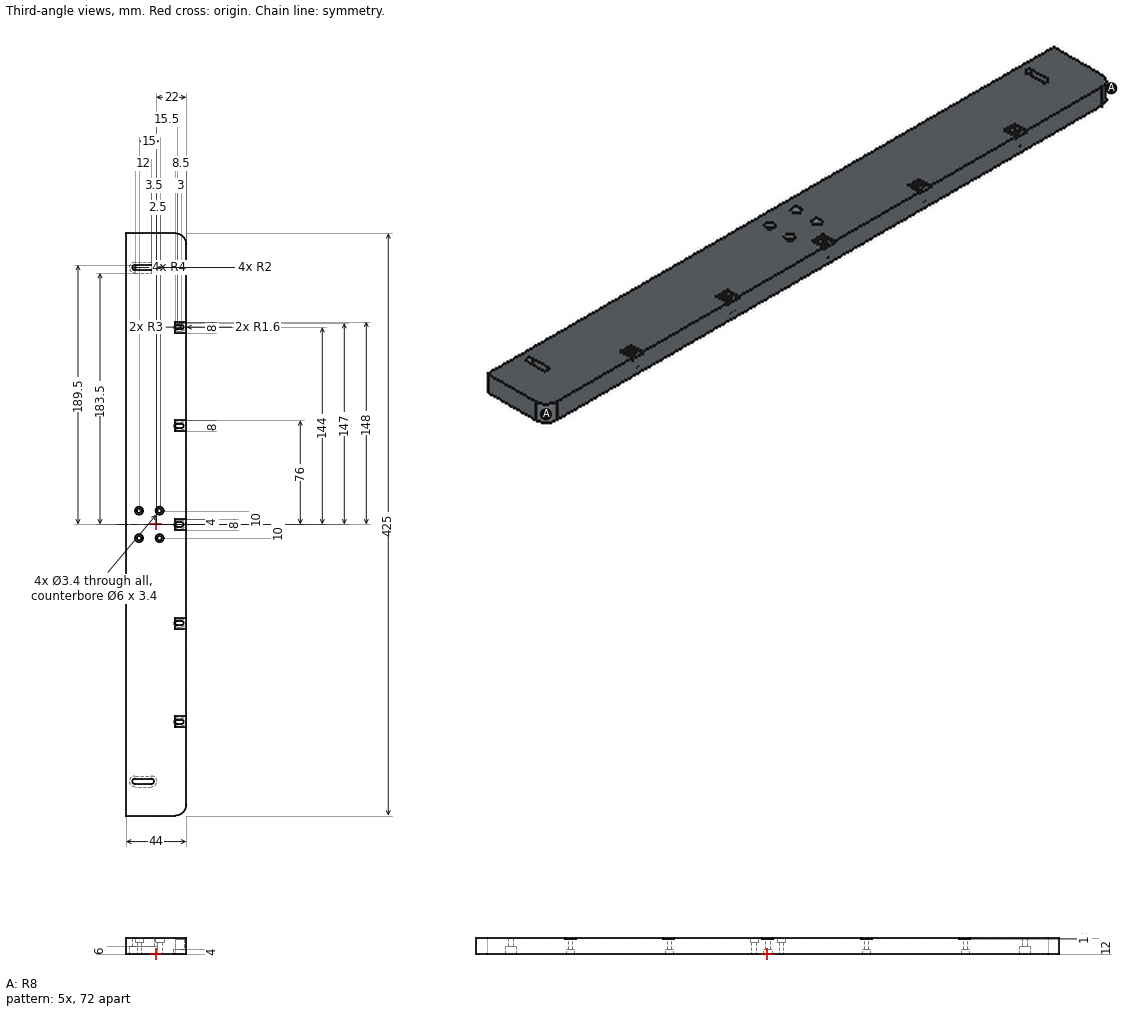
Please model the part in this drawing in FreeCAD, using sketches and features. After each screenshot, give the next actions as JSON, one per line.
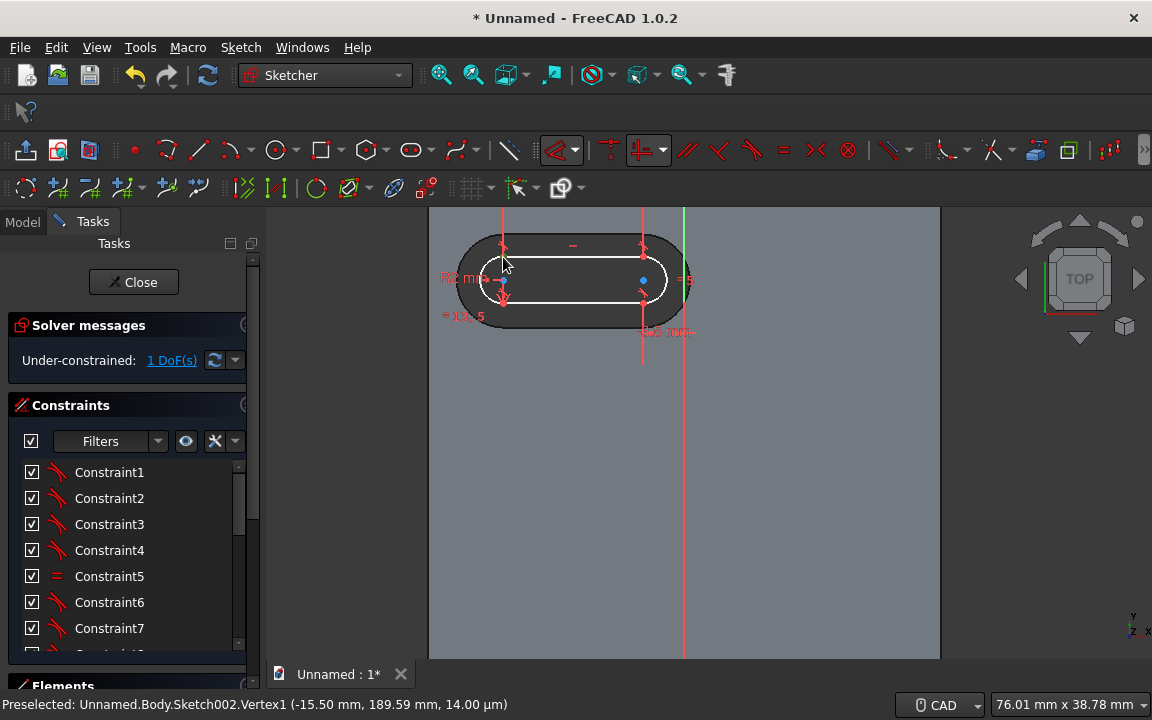
{"action": "key", "text": "i"}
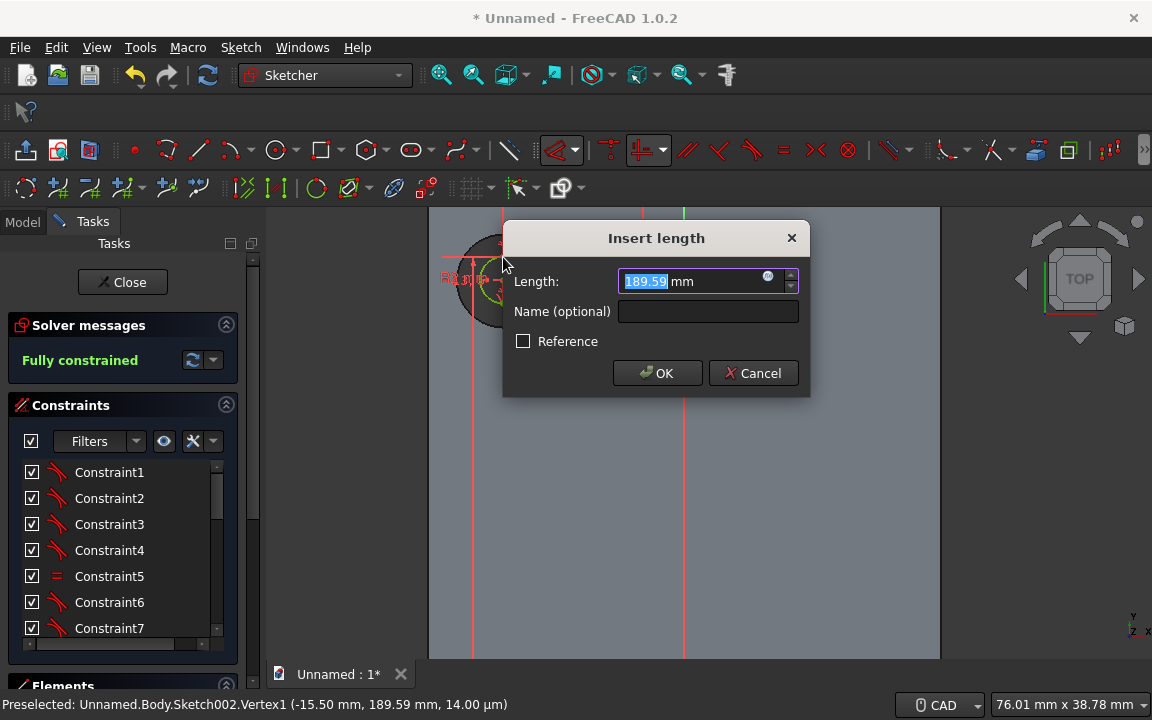
{"action": "type", "text": "189.5"}
{"action": "key", "text": "Return"}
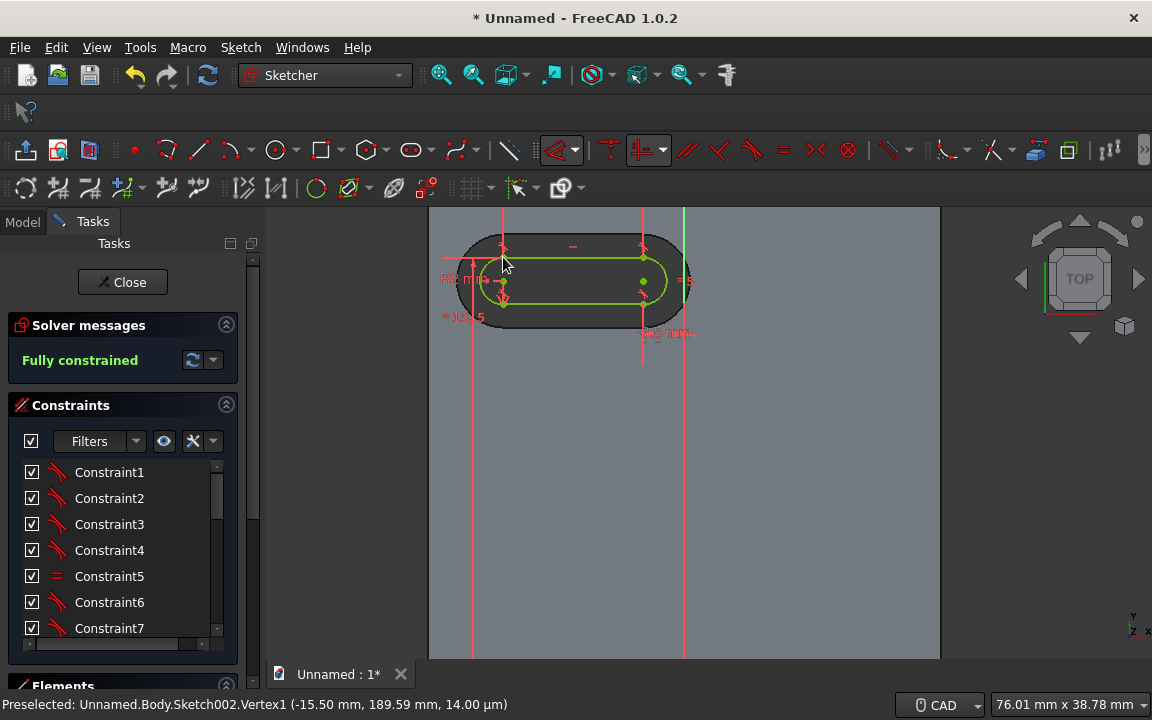
{"action": "left_click", "coordinate": [123, 282]}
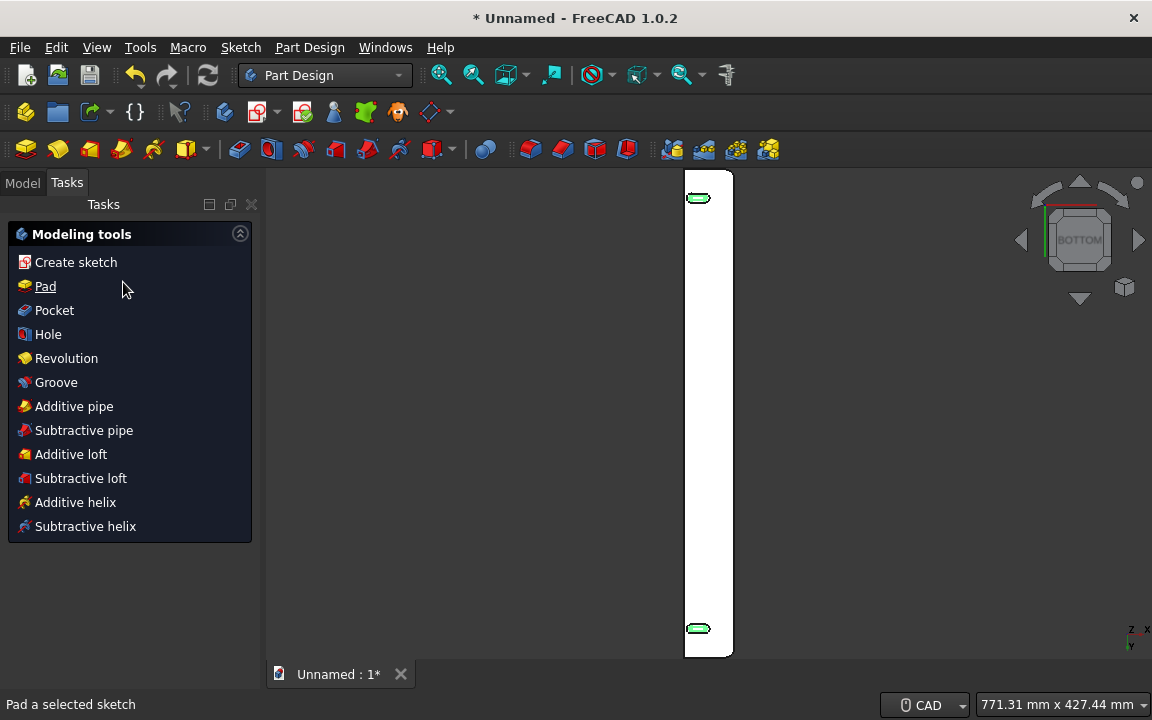
{"action": "left_click", "coordinate": [240, 150]}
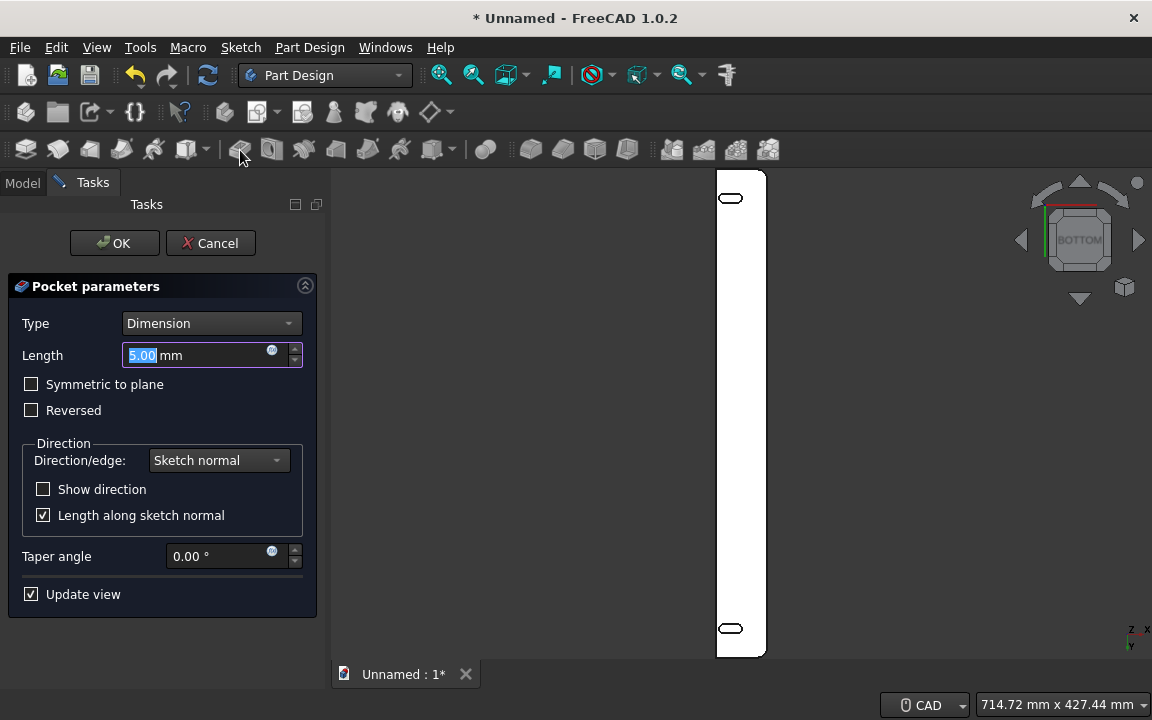
{"action": "left_click", "coordinate": [212, 324]}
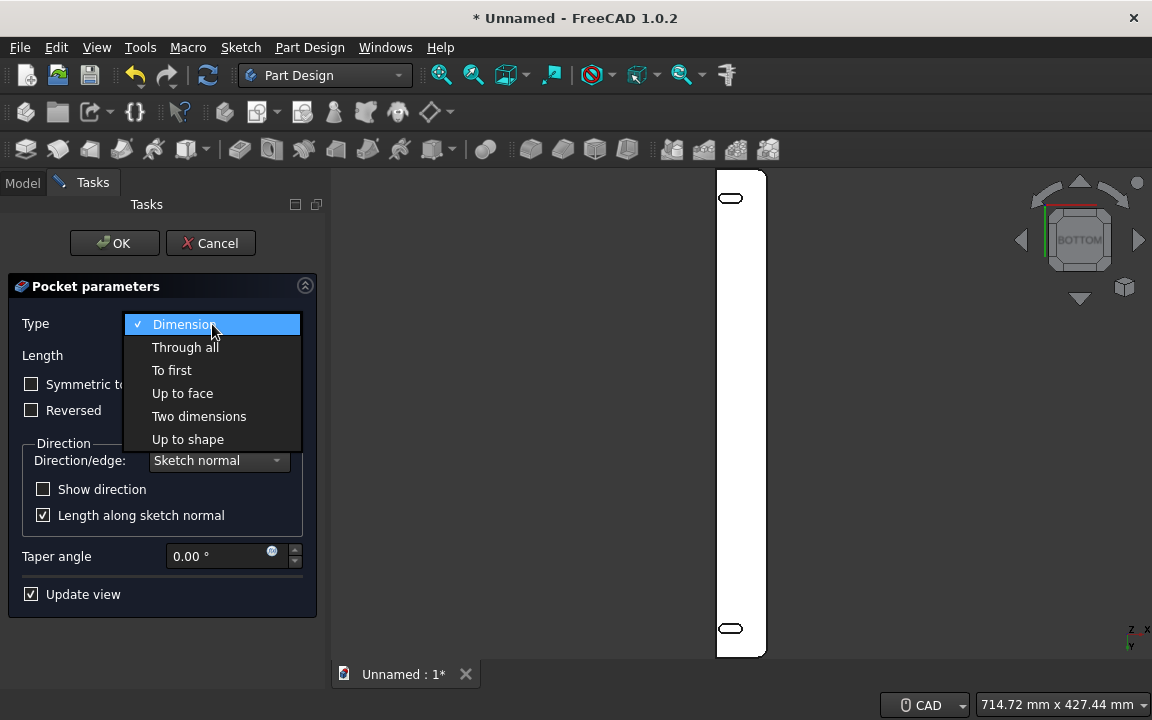
{"action": "left_click", "coordinate": [212, 348]}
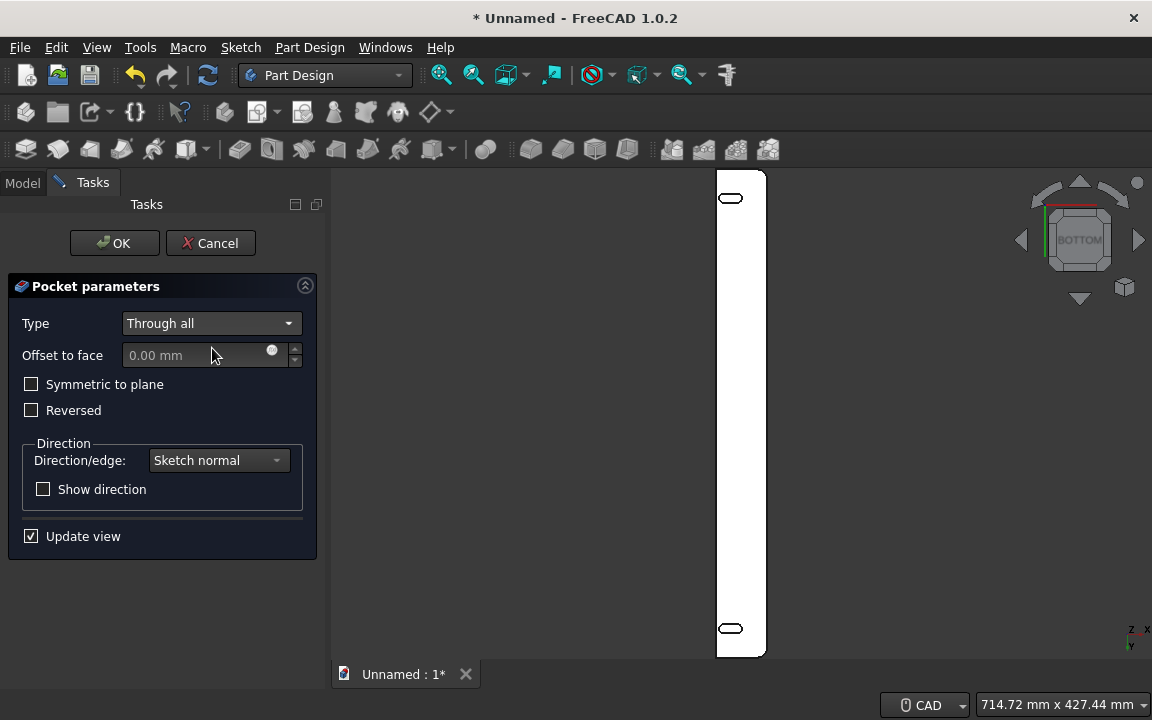
{"action": "left_click", "coordinate": [30, 410]}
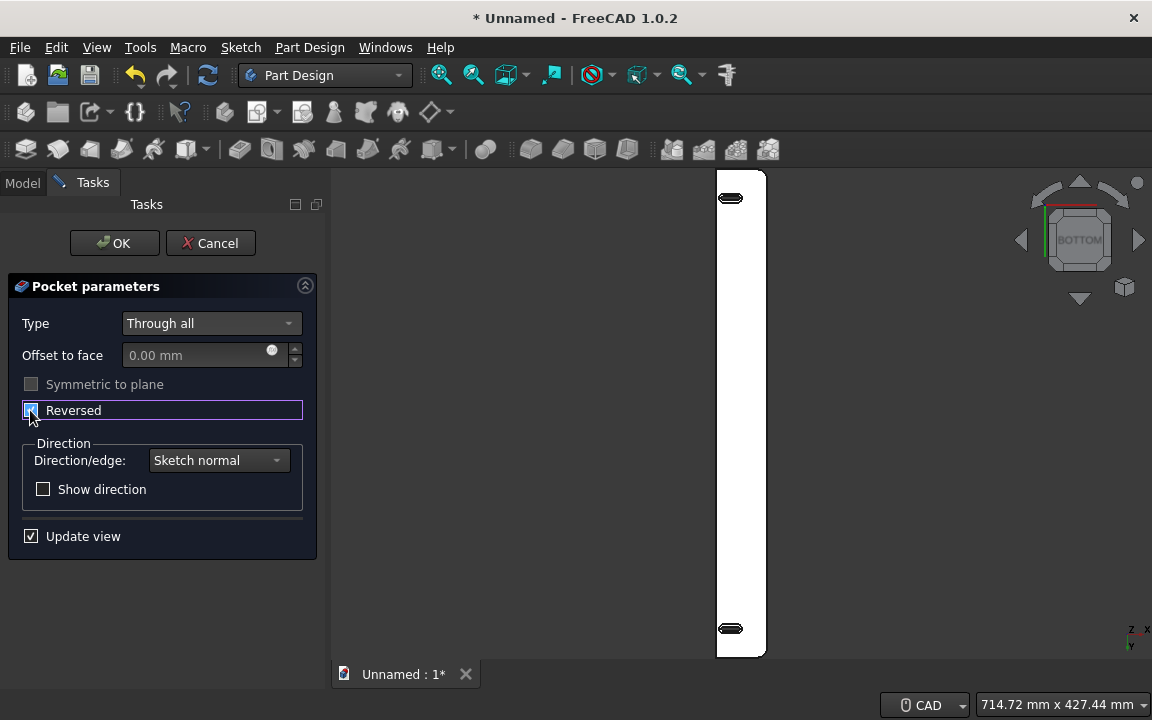
{"action": "left_click", "coordinate": [115, 243]}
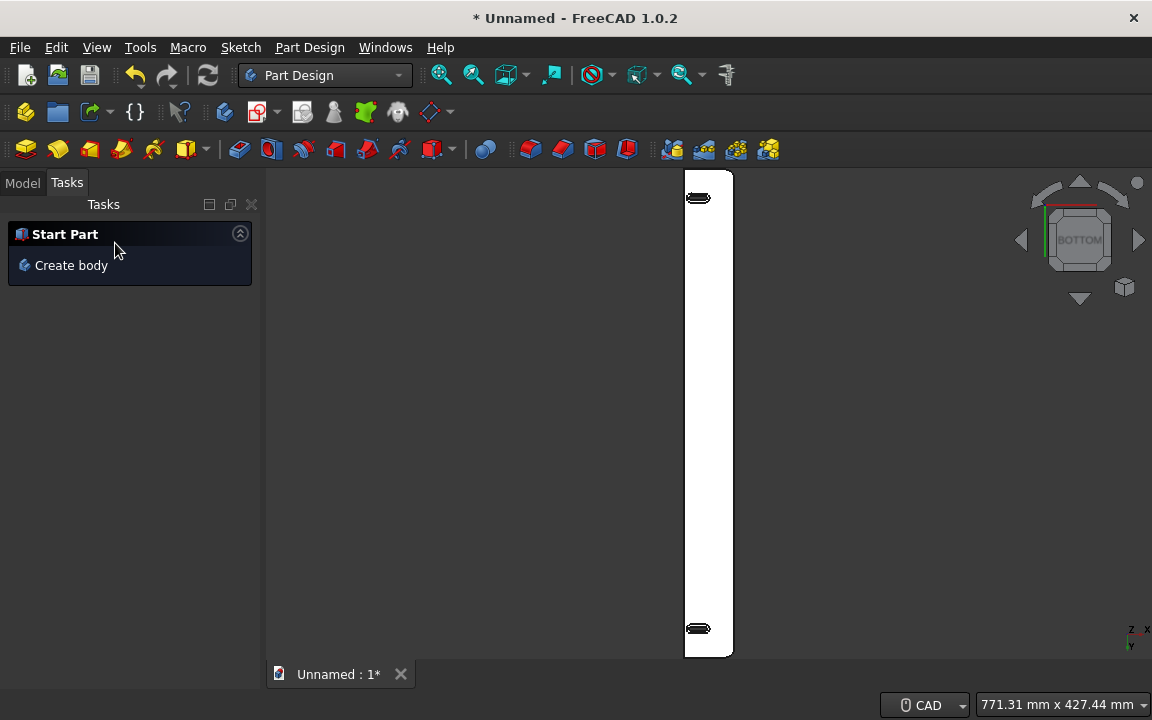
{"action": "key", "text": "0"}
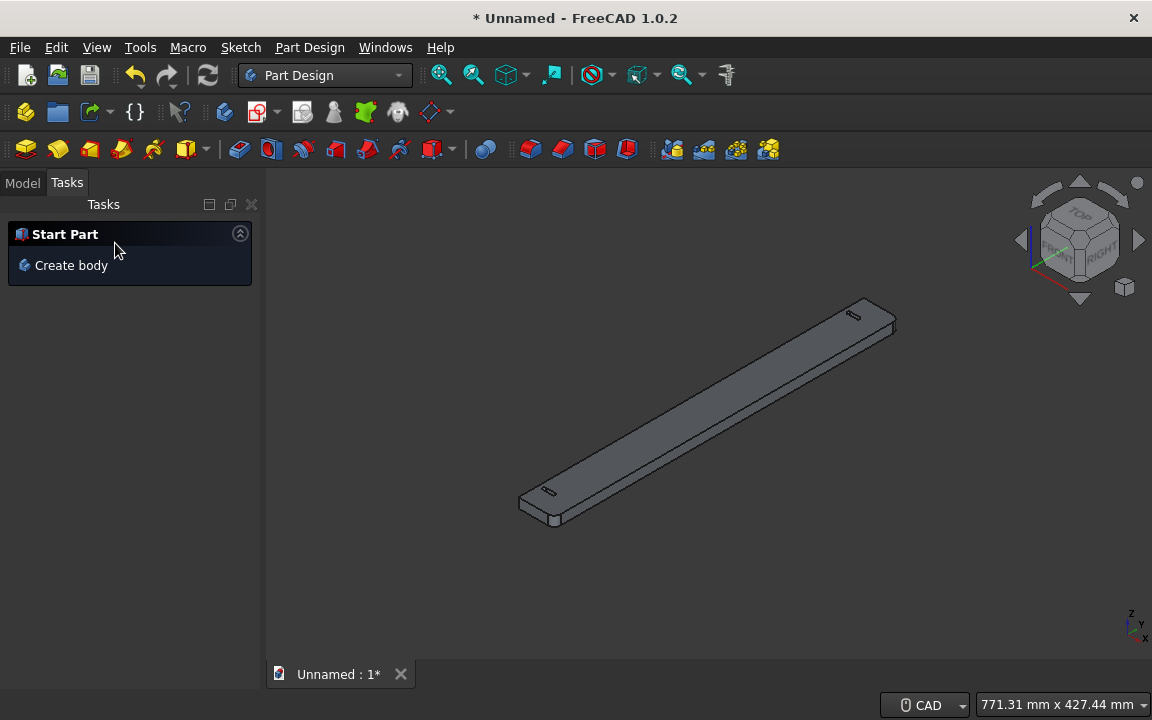
{"action": "left_click", "coordinate": [808, 350]}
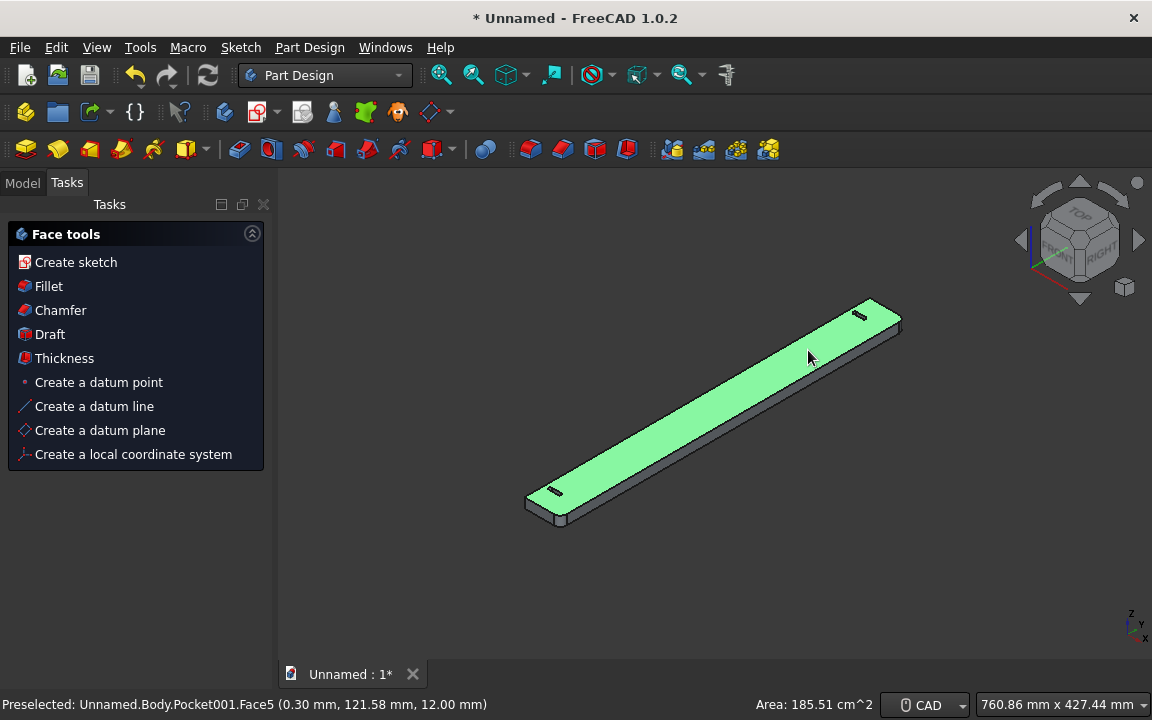
{"action": "left_click", "coordinate": [258, 112]}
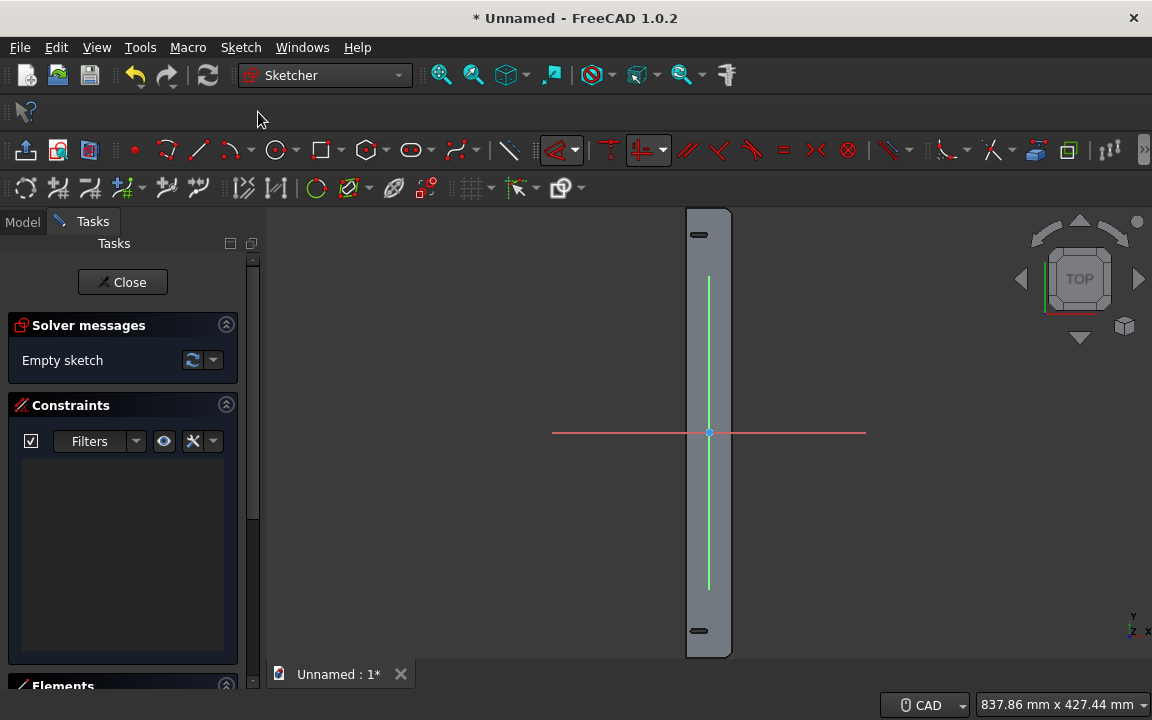
{"action": "key", "text": "g r"}